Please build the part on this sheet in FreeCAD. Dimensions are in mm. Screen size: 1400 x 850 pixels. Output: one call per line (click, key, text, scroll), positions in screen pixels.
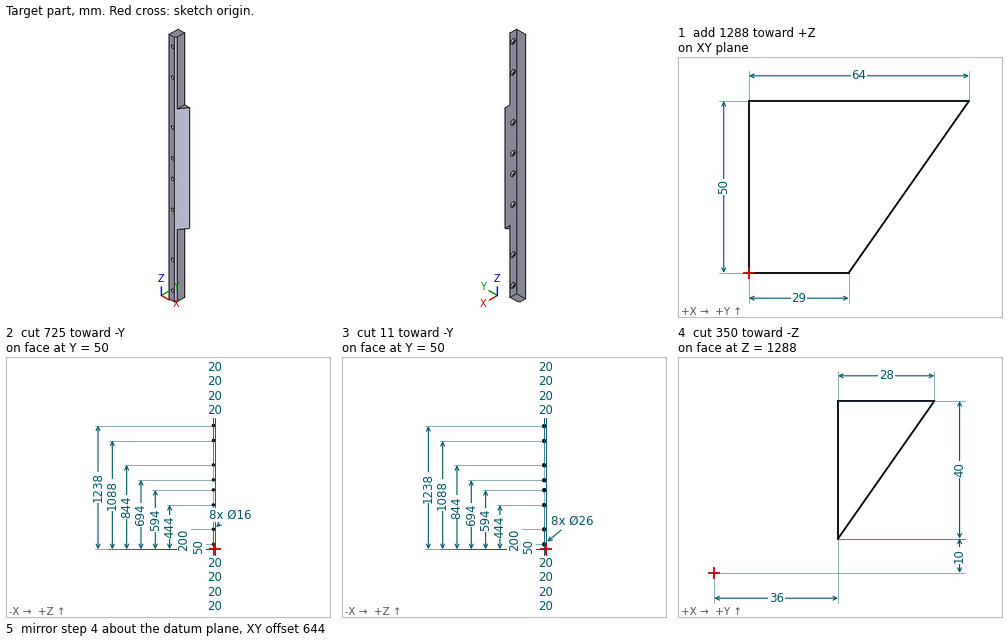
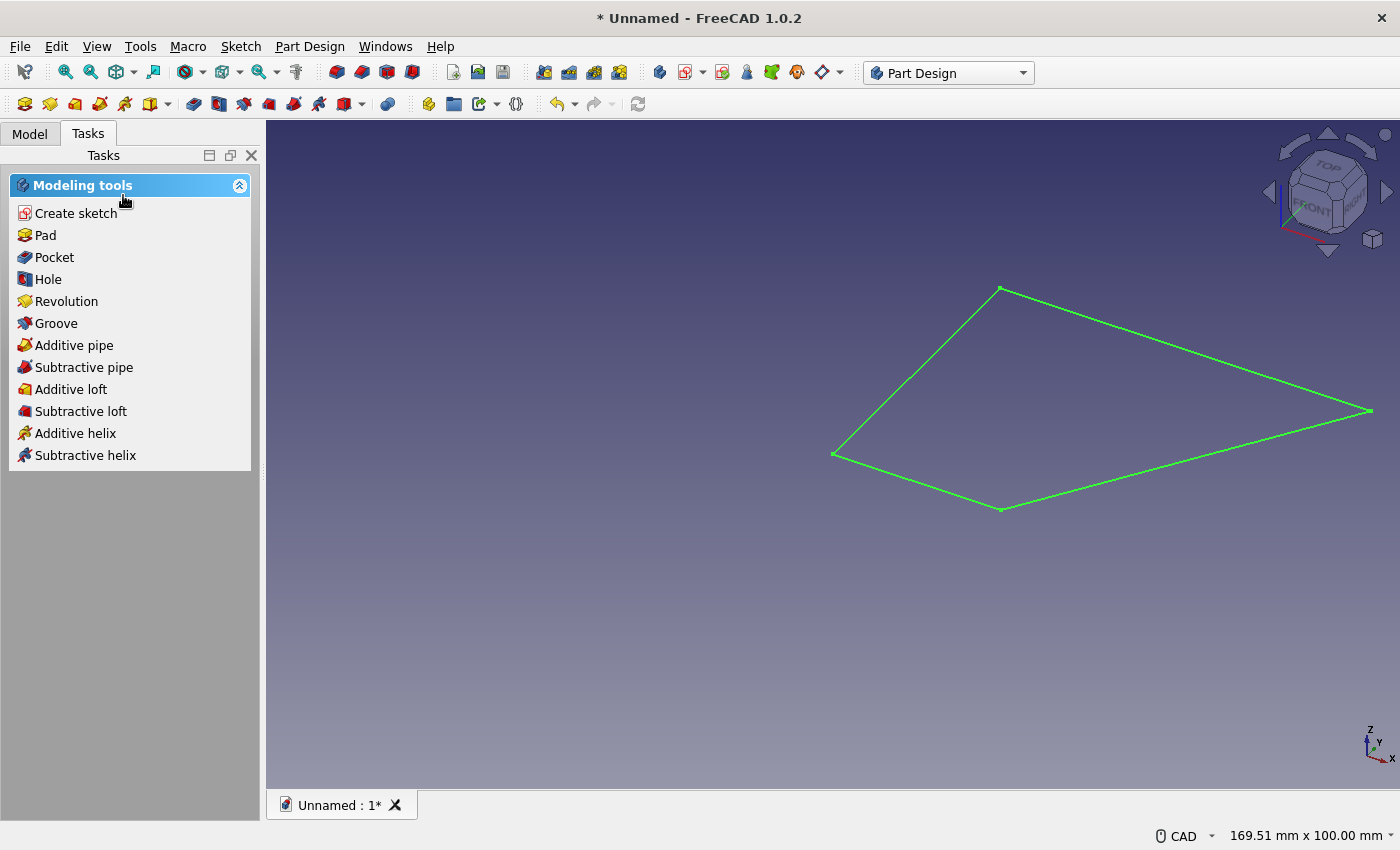
click(25, 104)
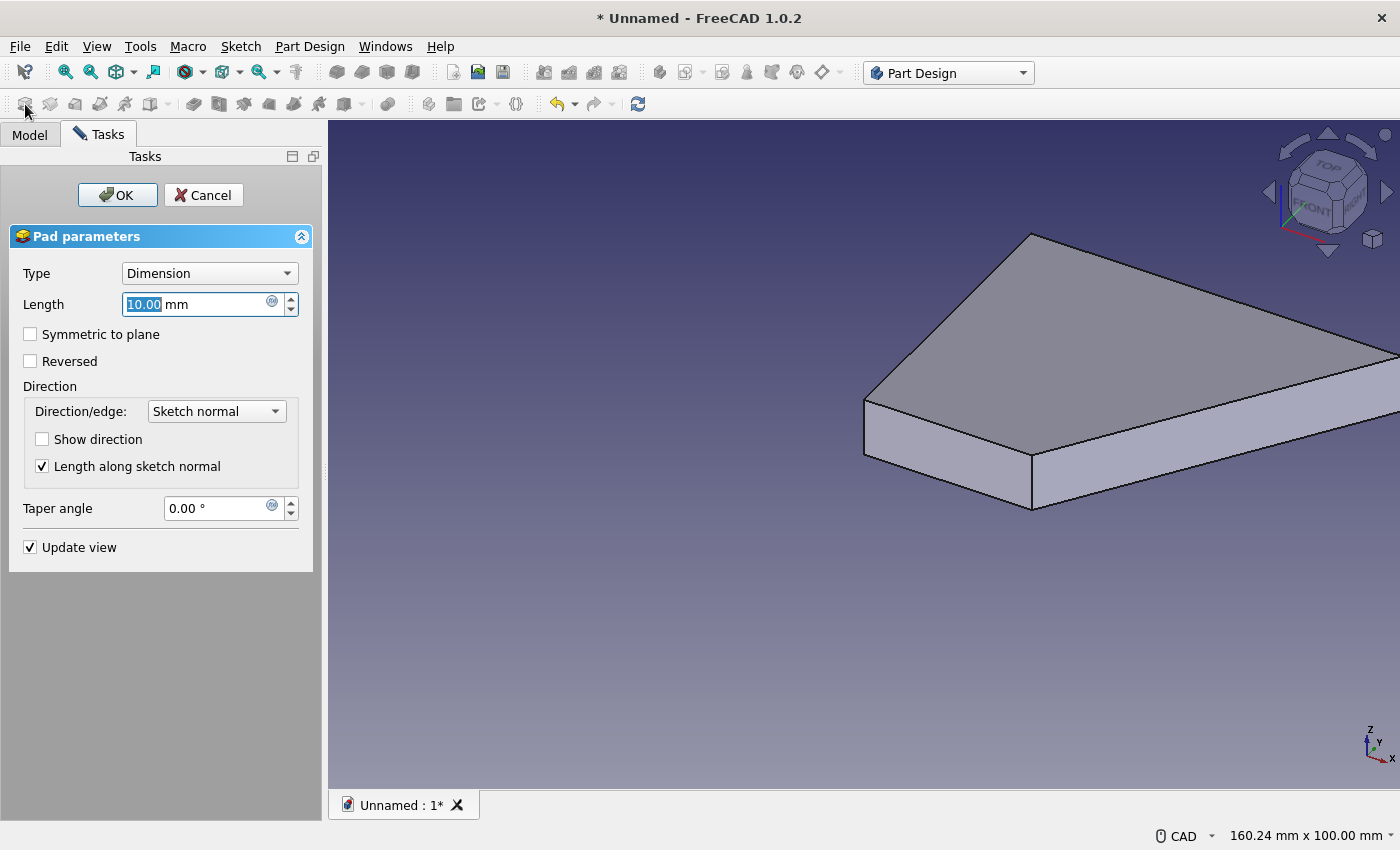
text(1288)
key(Tab)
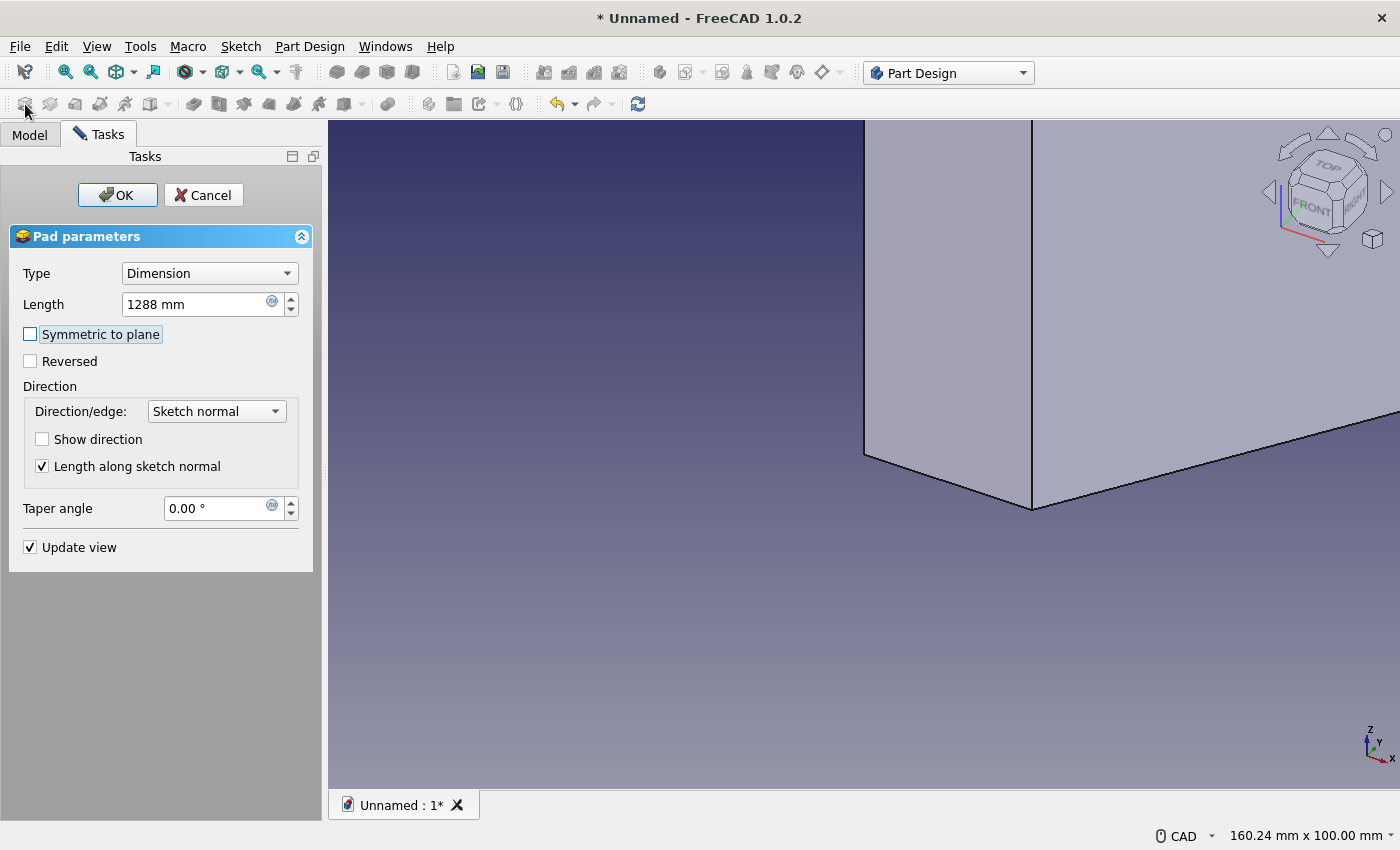
click(118, 195)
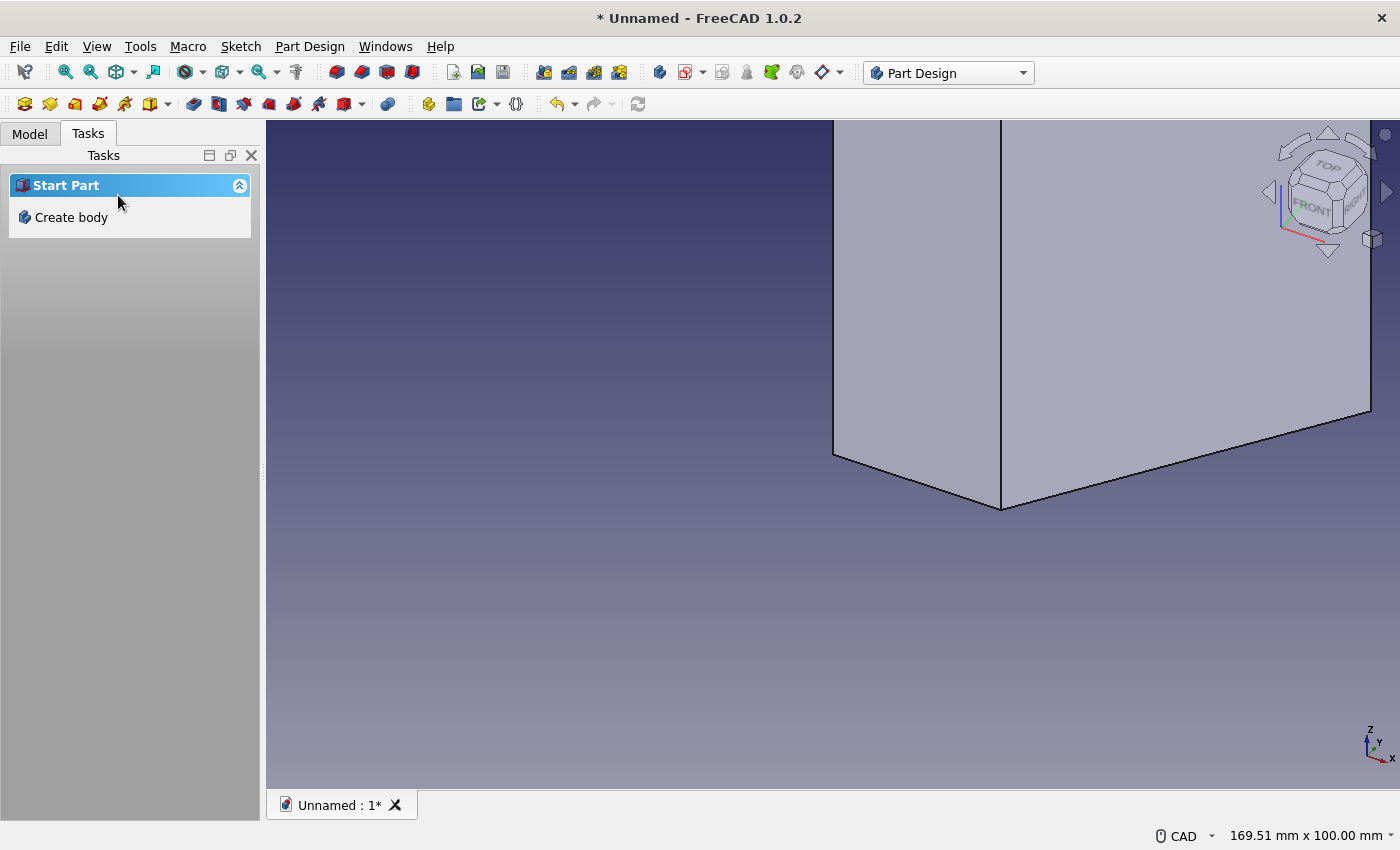
key(v)
key(f)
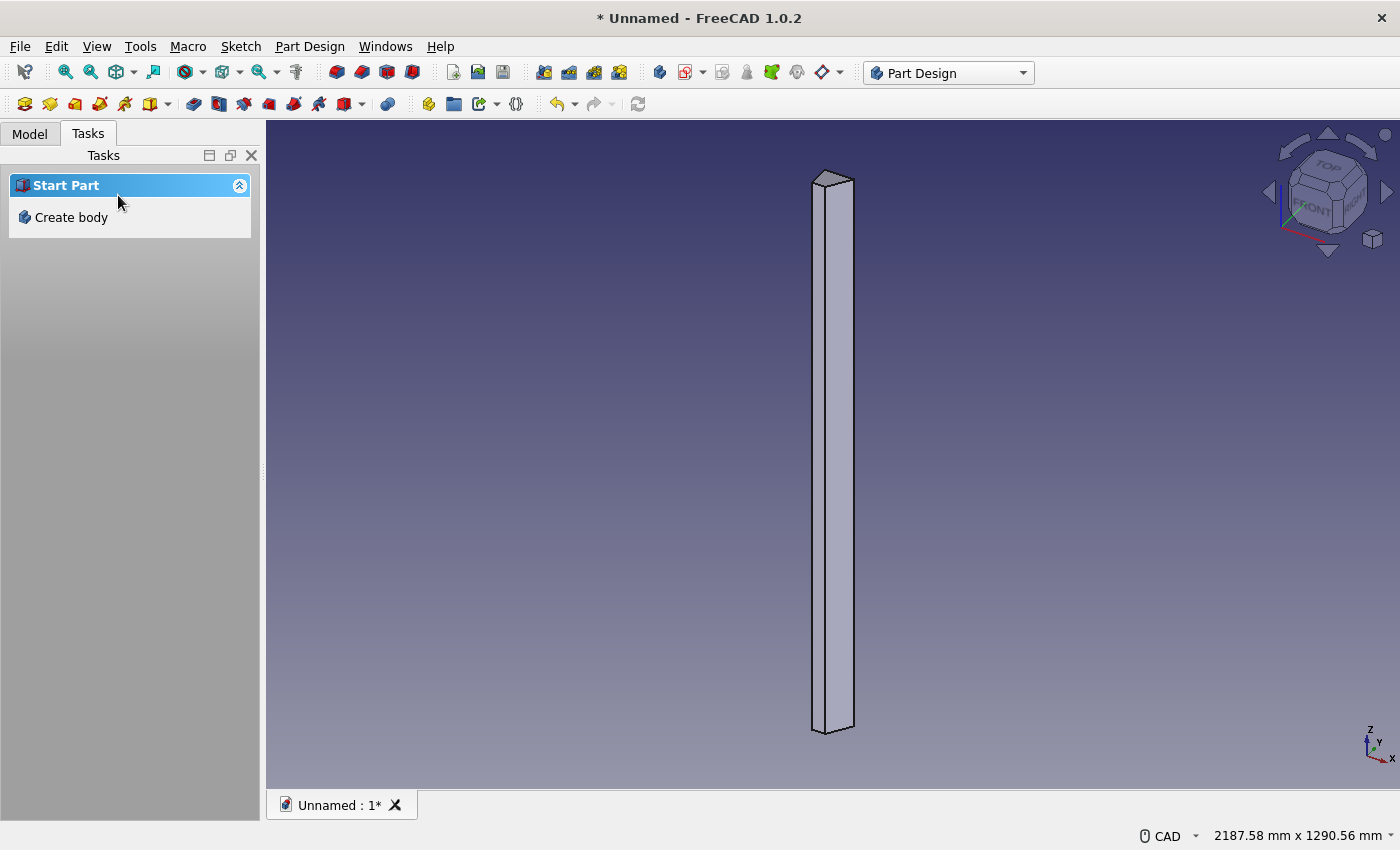
key(4)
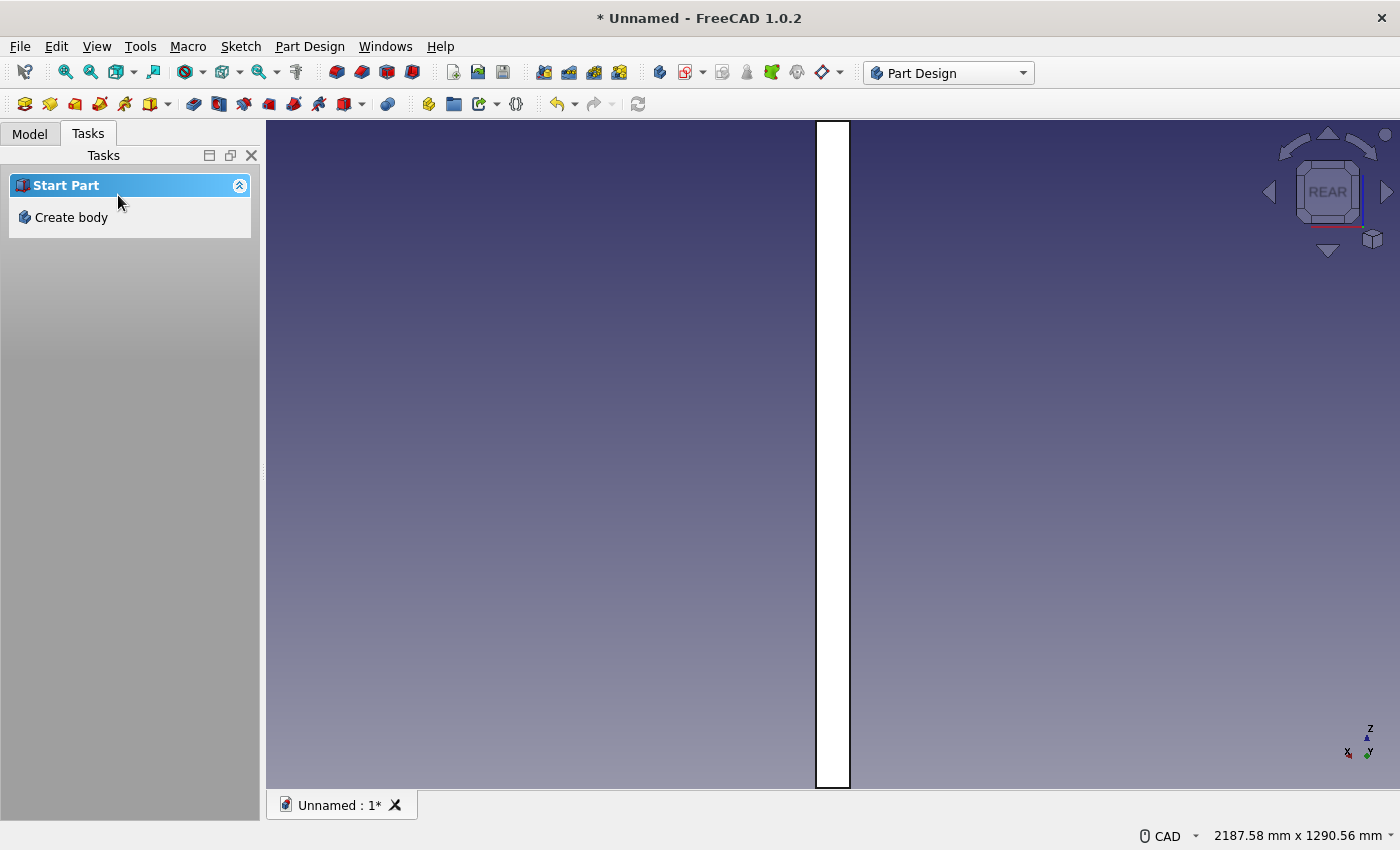
click(833, 167)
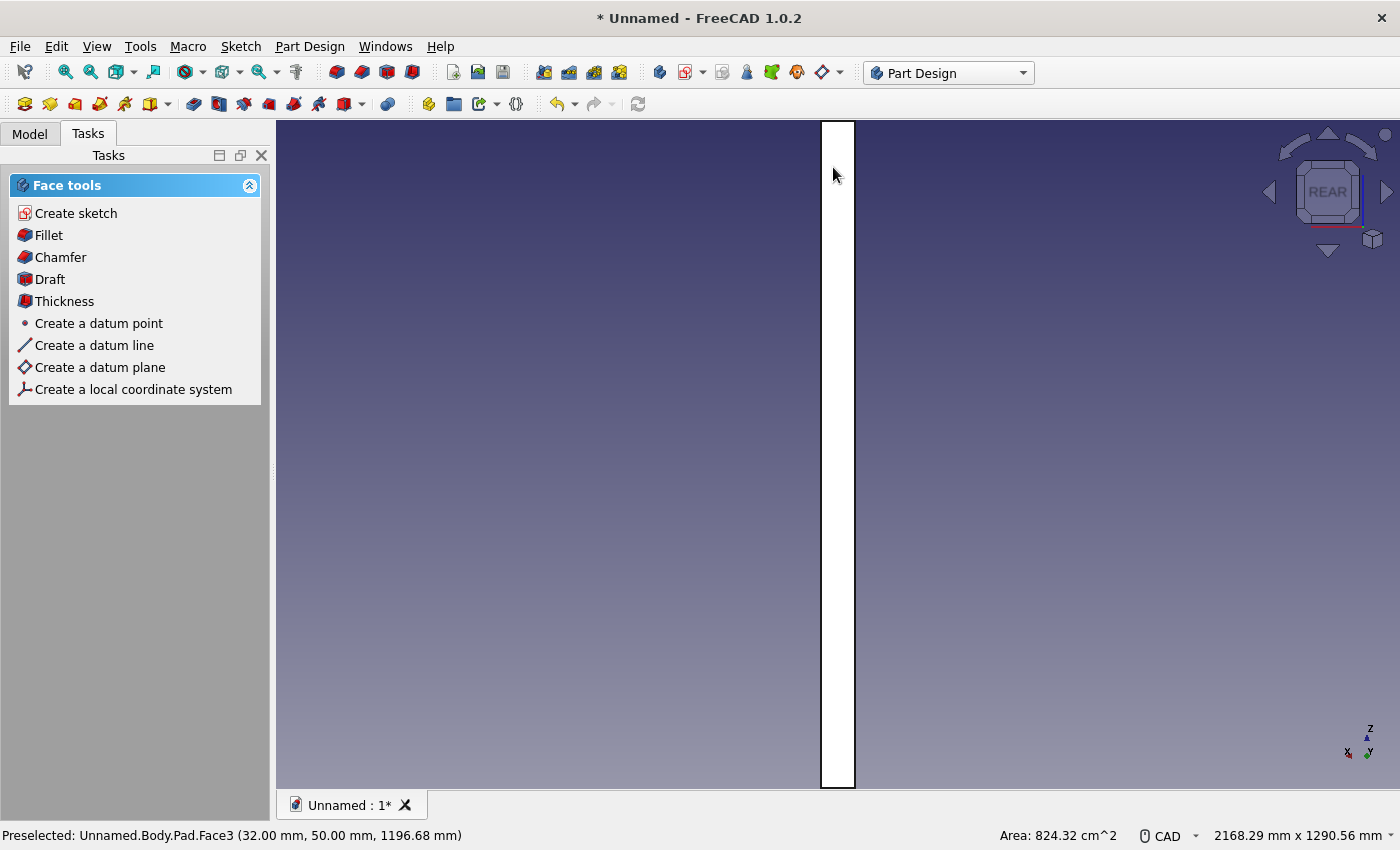
click(684, 72)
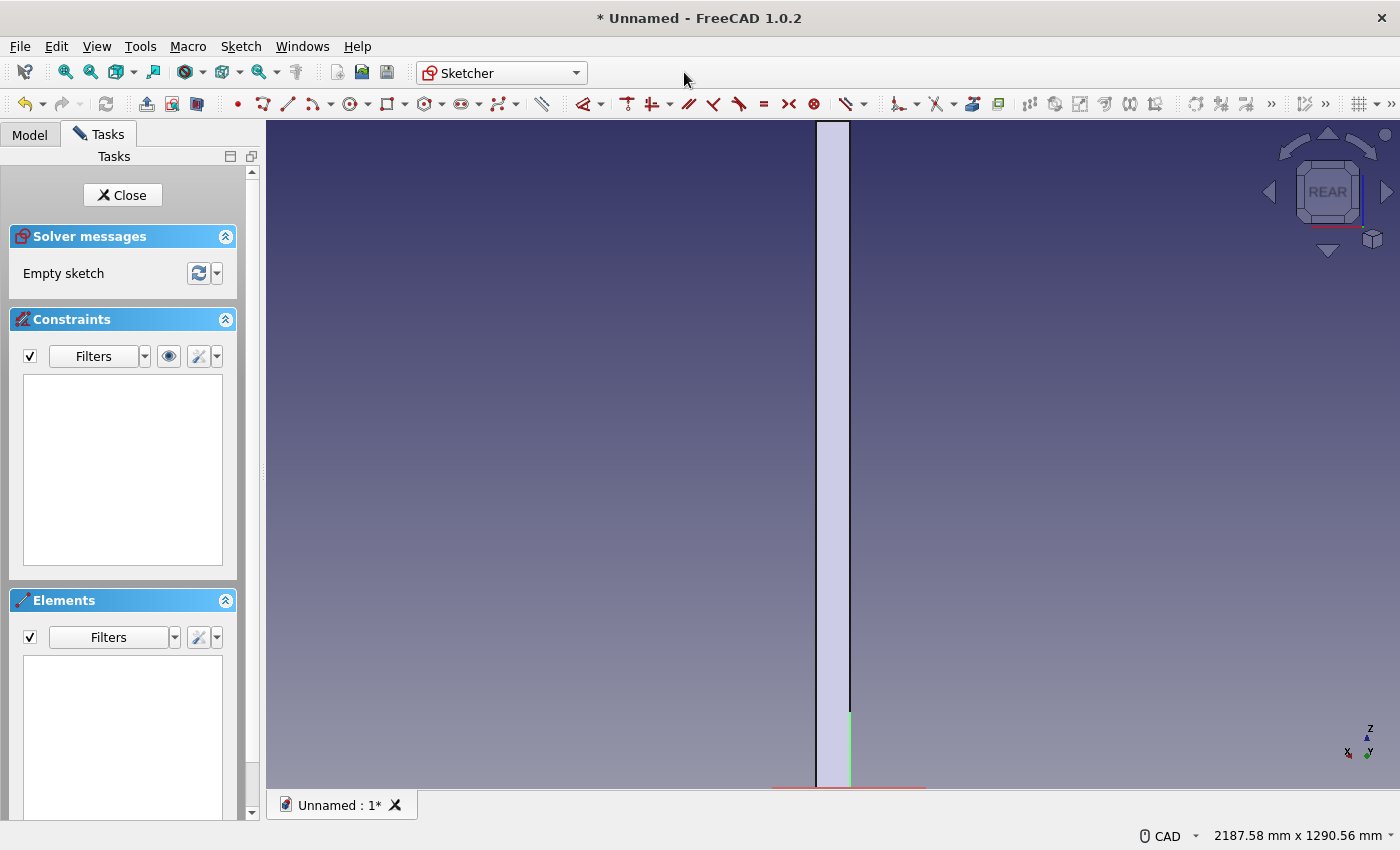
scroll(606, 432, down, 2)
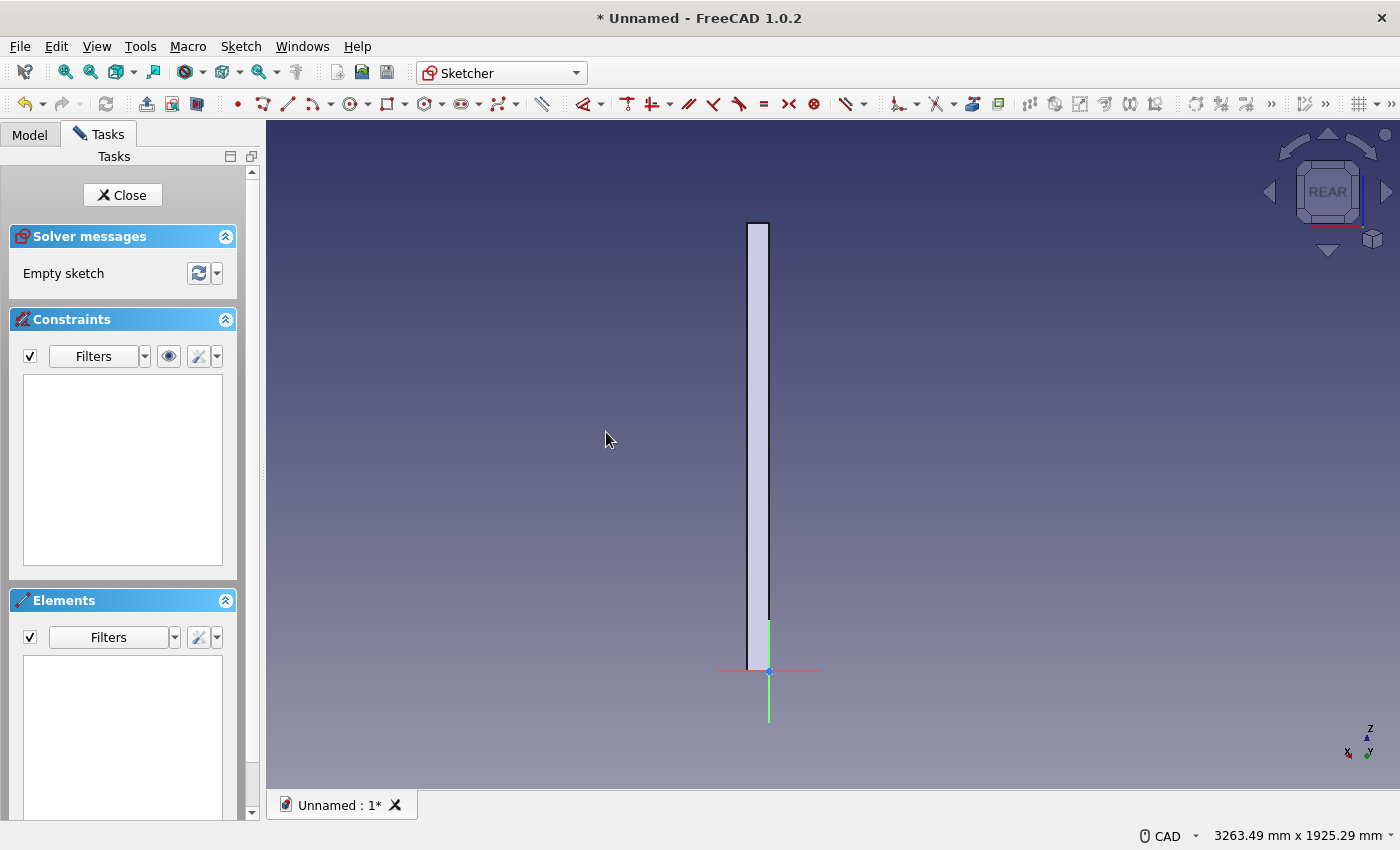
key(g)
key(c)